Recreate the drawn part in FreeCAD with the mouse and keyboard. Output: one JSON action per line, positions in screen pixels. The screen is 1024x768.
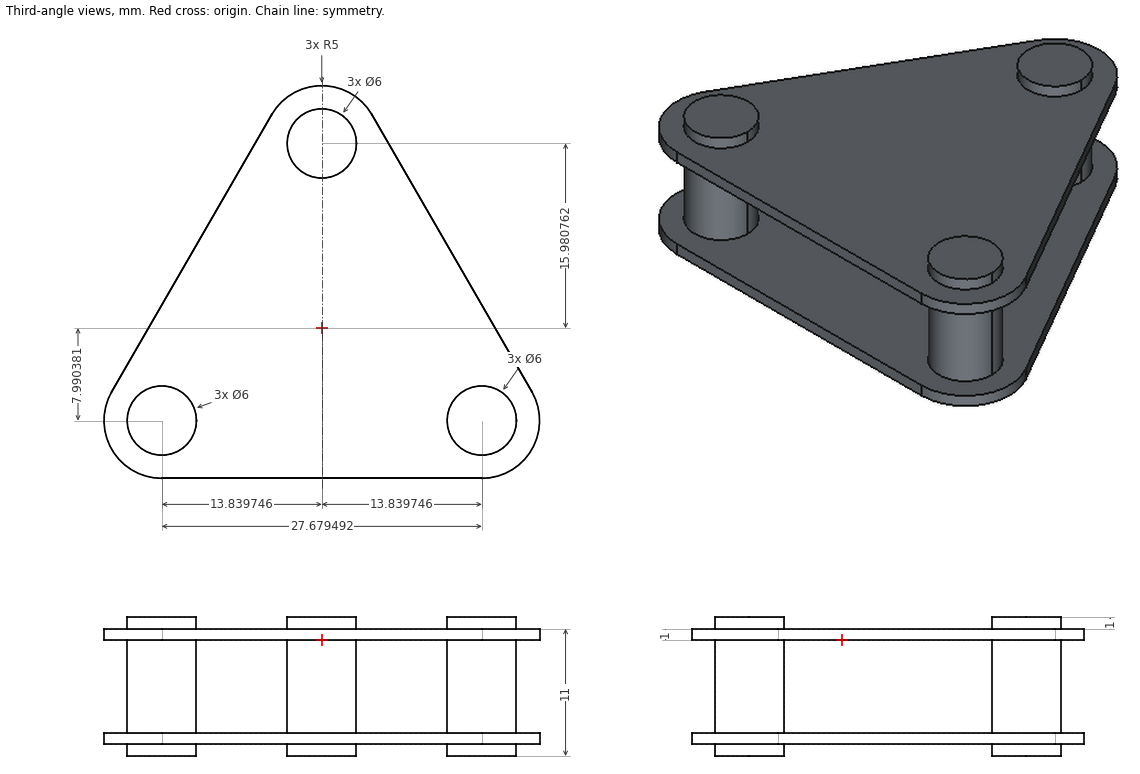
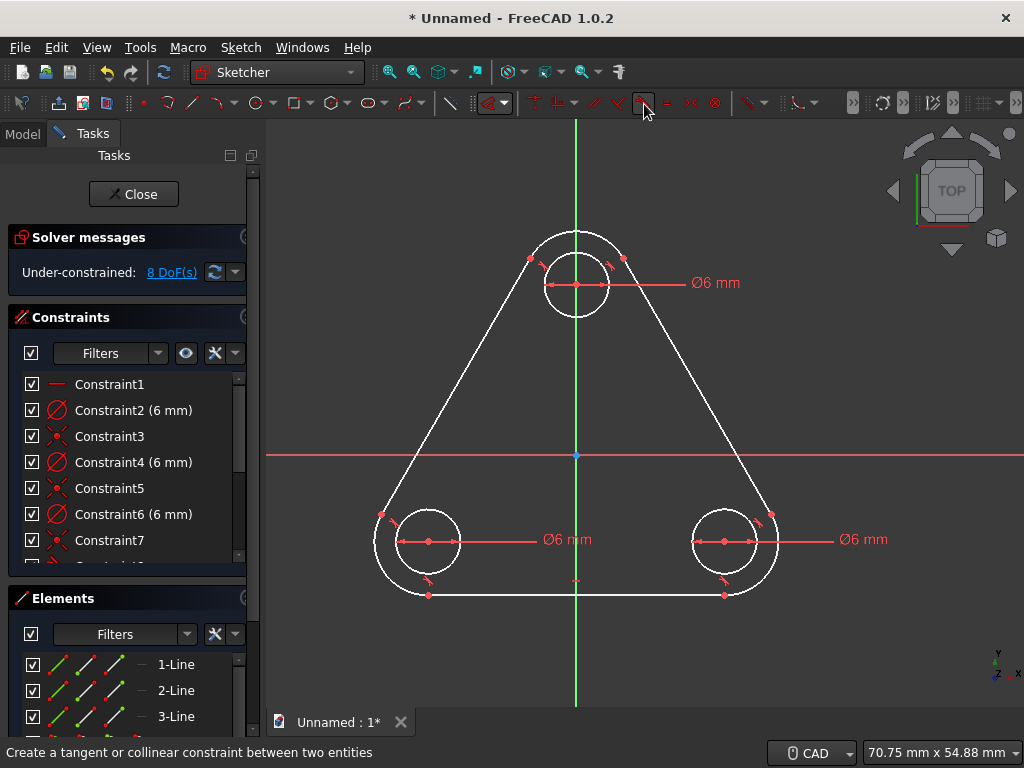
{"action": "left_click", "coordinate": [599, 236]}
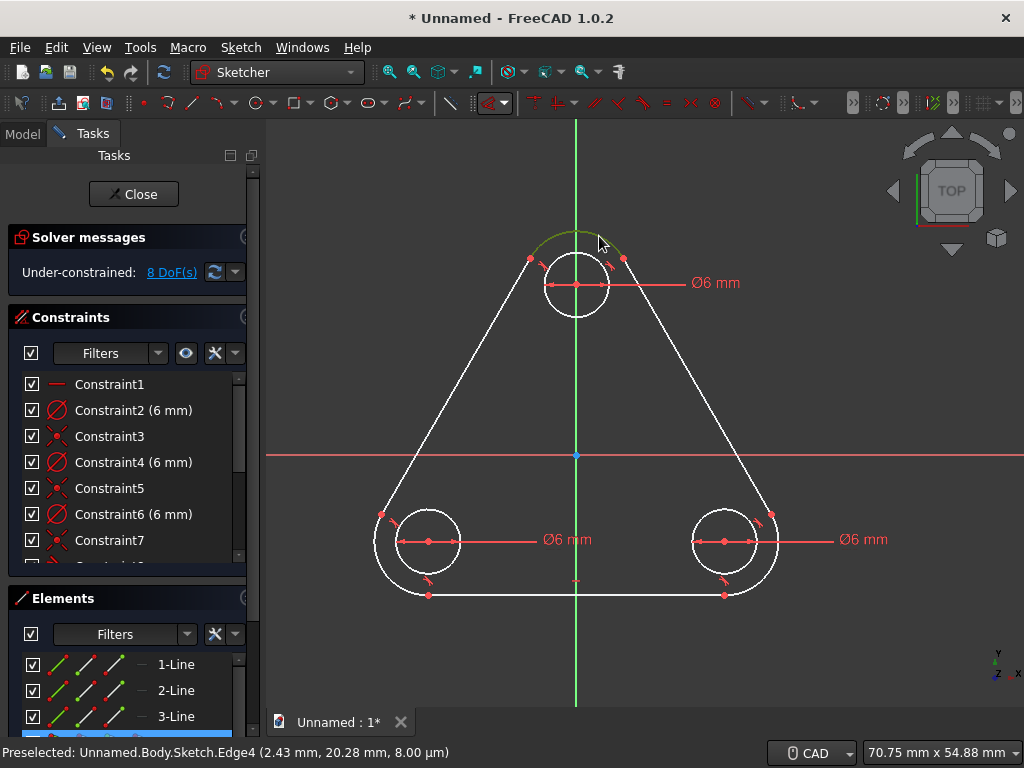
{"action": "left_click", "coordinate": [375, 547]}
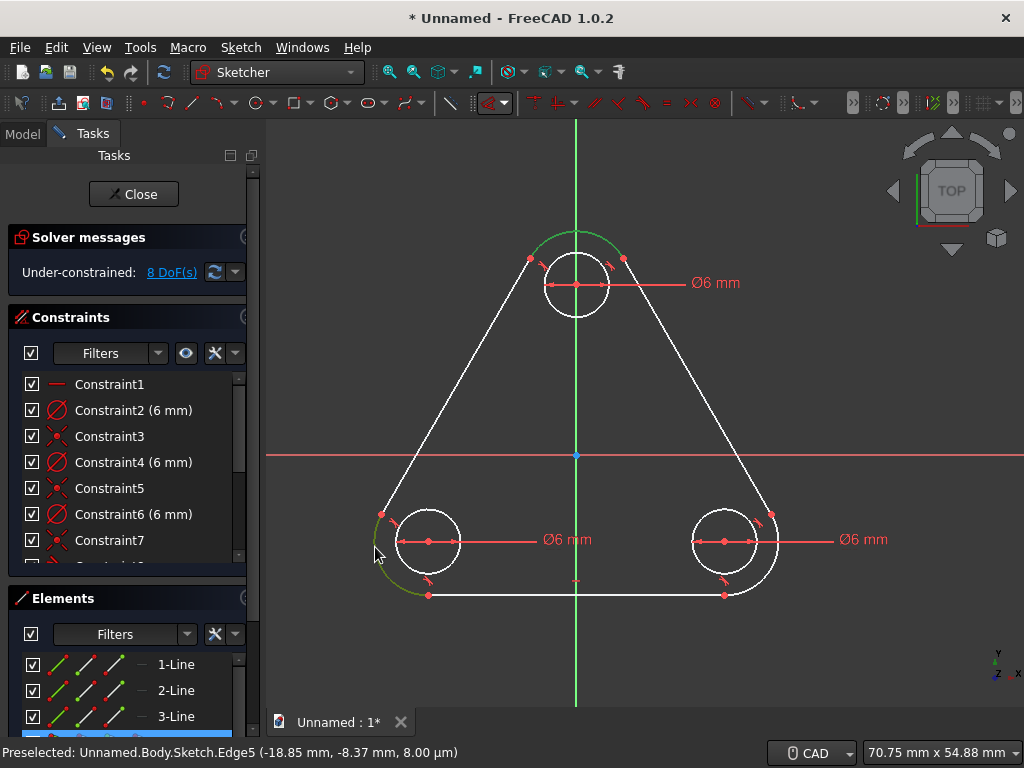
{"action": "left_click", "coordinate": [756, 585]}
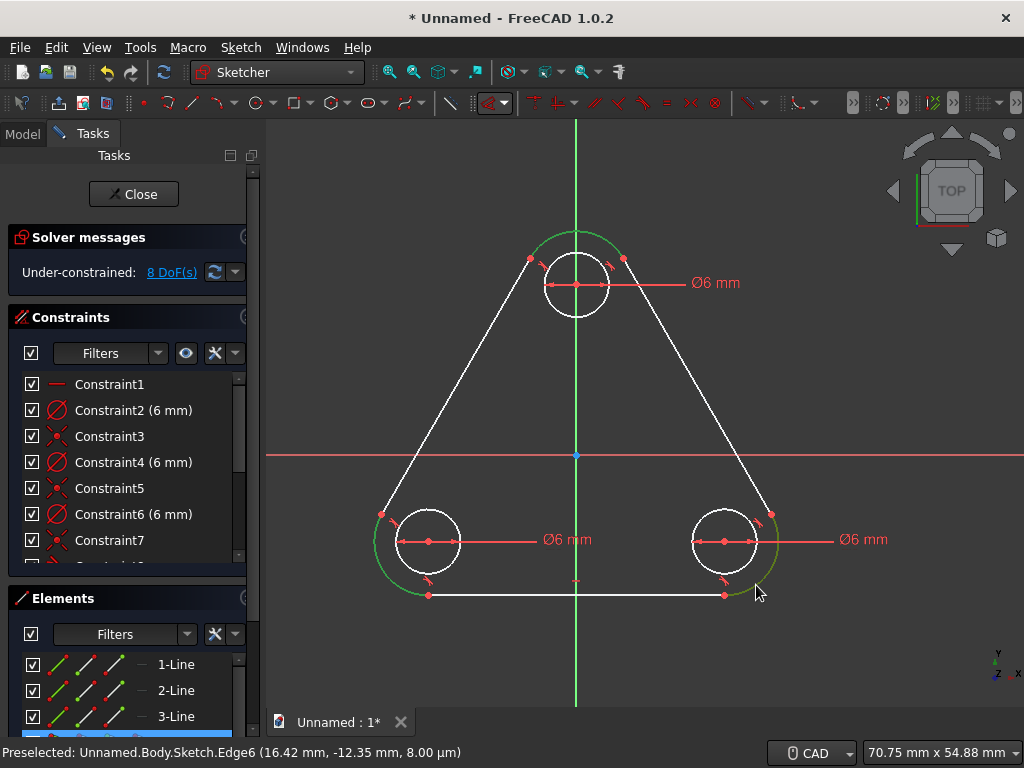
{"action": "left_click", "coordinate": [668, 104]}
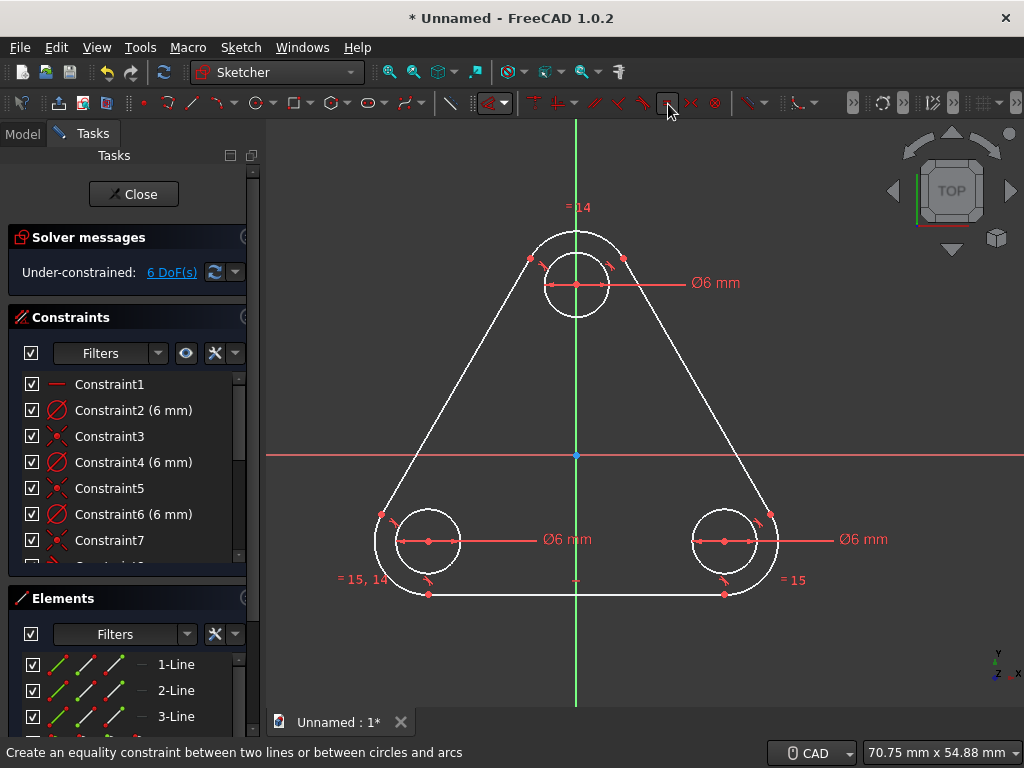
{"action": "left_click", "coordinate": [577, 285]}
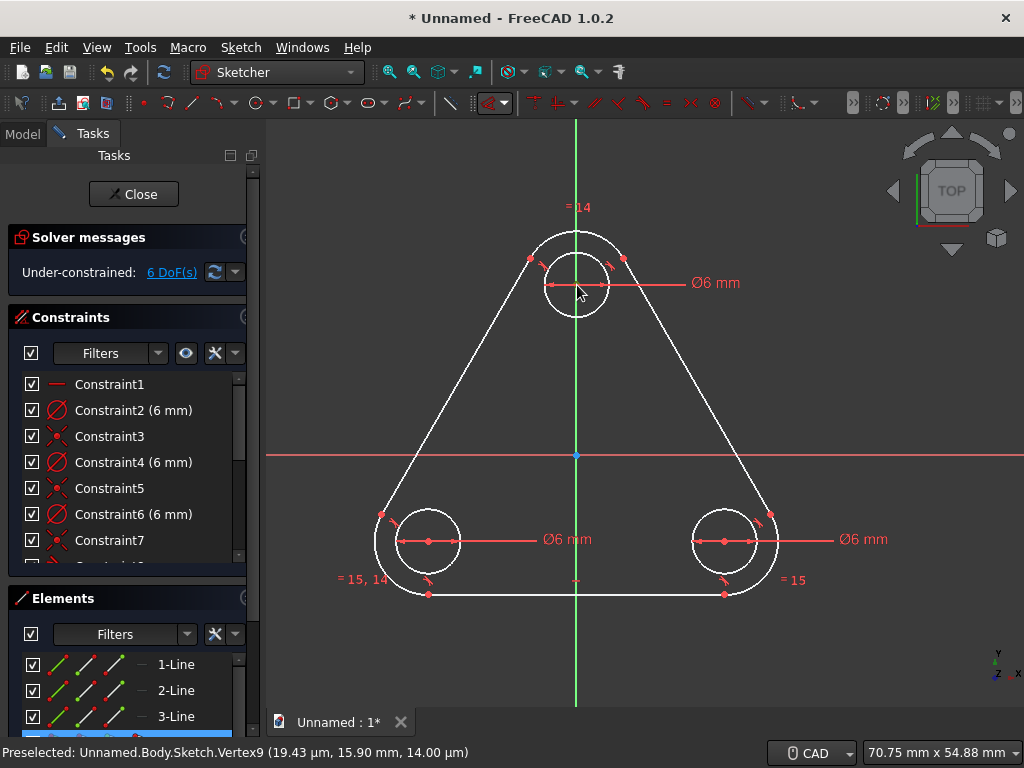
{"action": "left_click", "coordinate": [576, 641]}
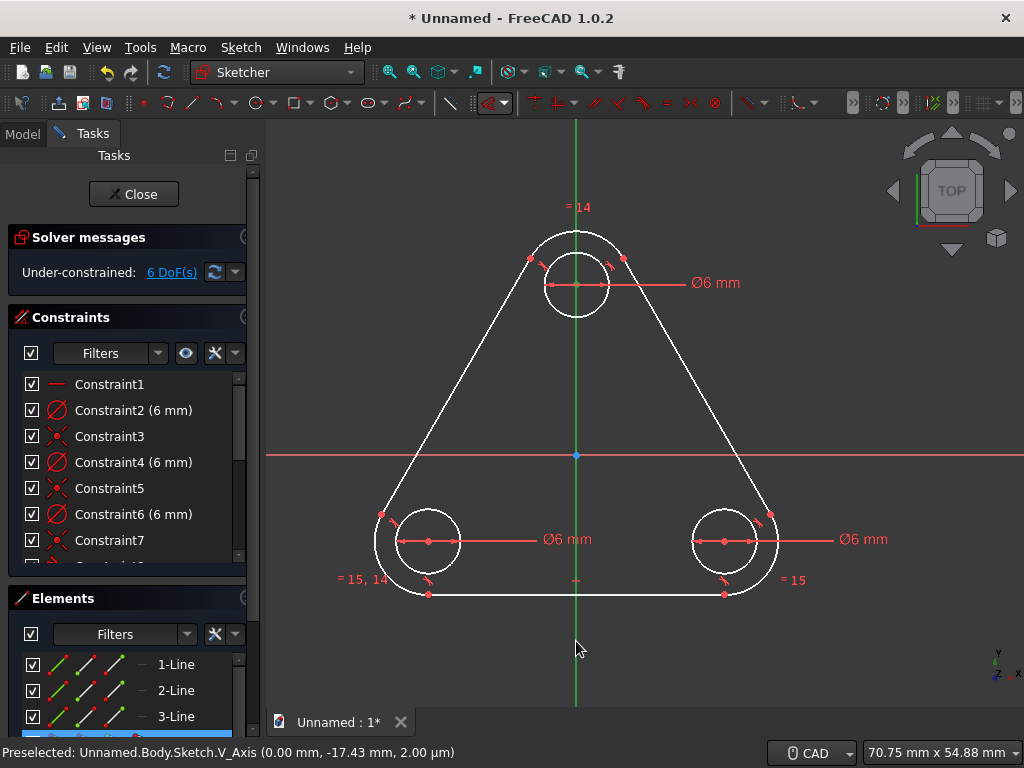
{"action": "left_click", "coordinate": [534, 104]}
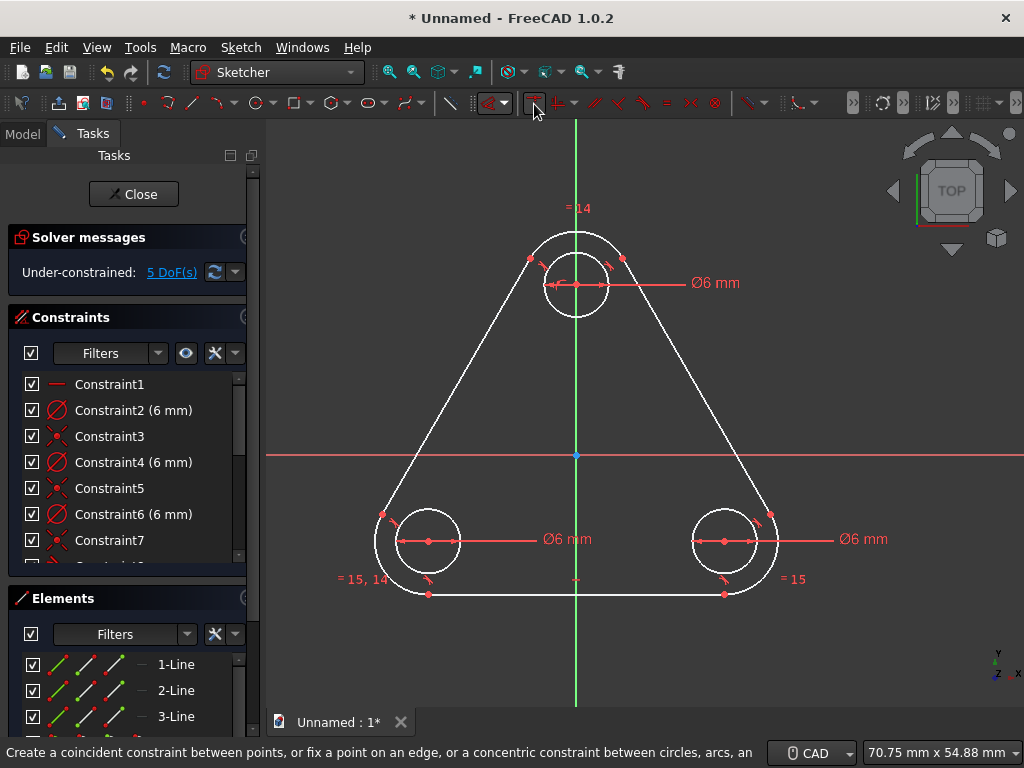
{"action": "left_click", "coordinate": [598, 236]}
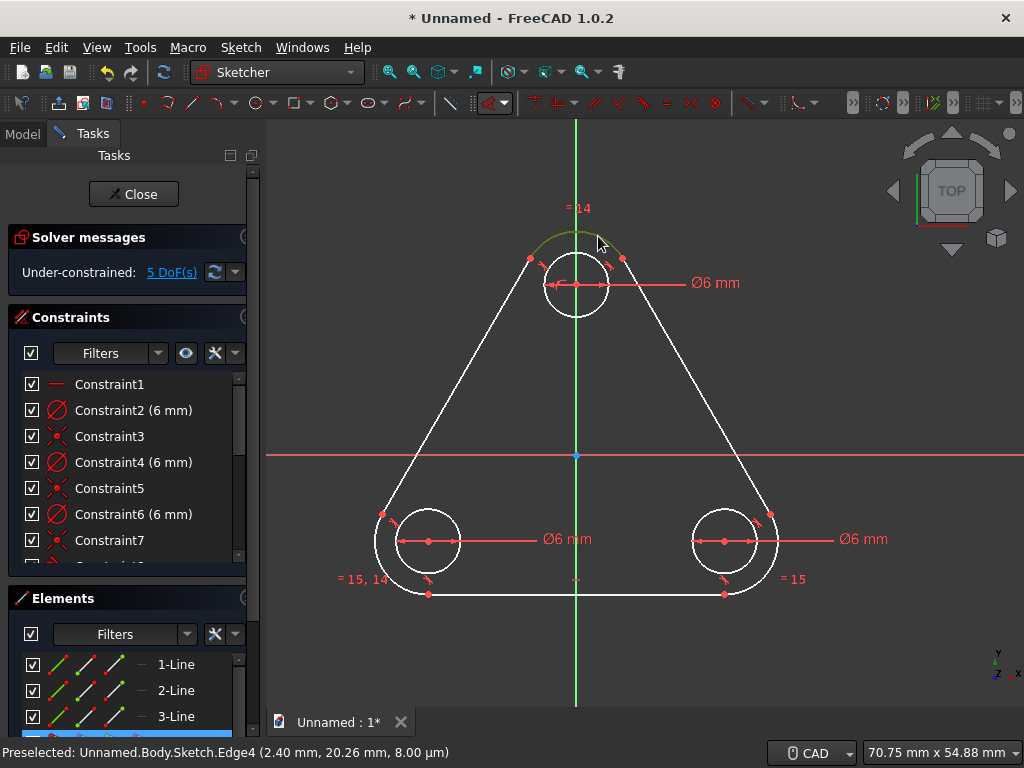
{"action": "left_click", "coordinate": [506, 104]}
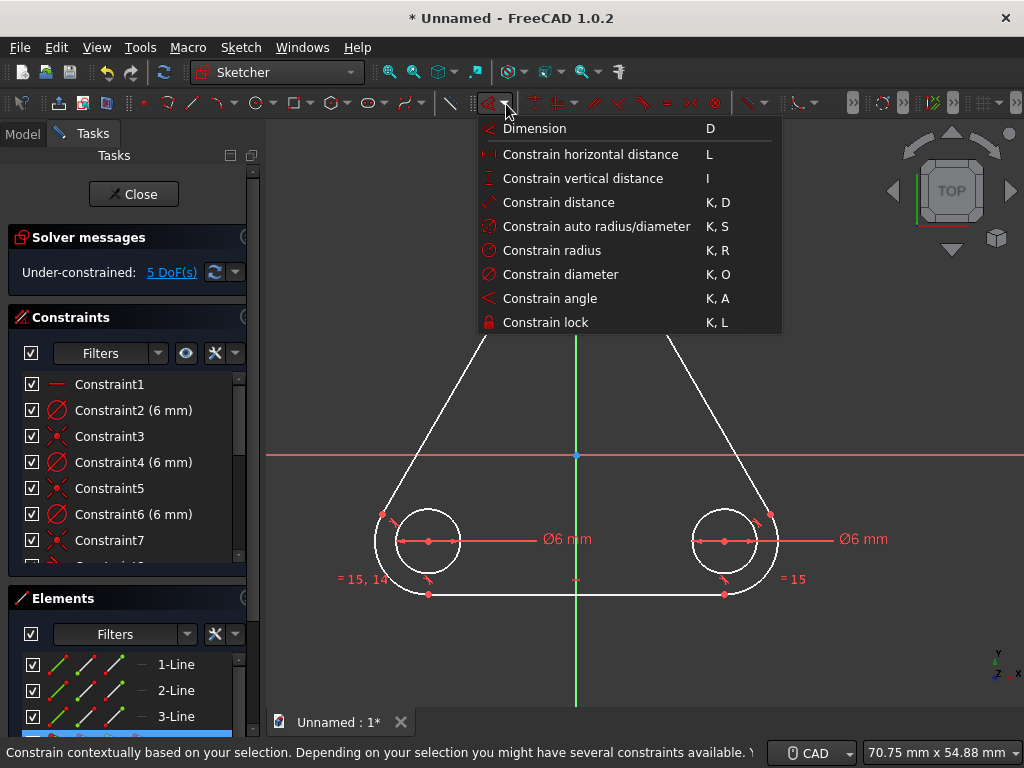
{"action": "left_click", "coordinate": [630, 250]}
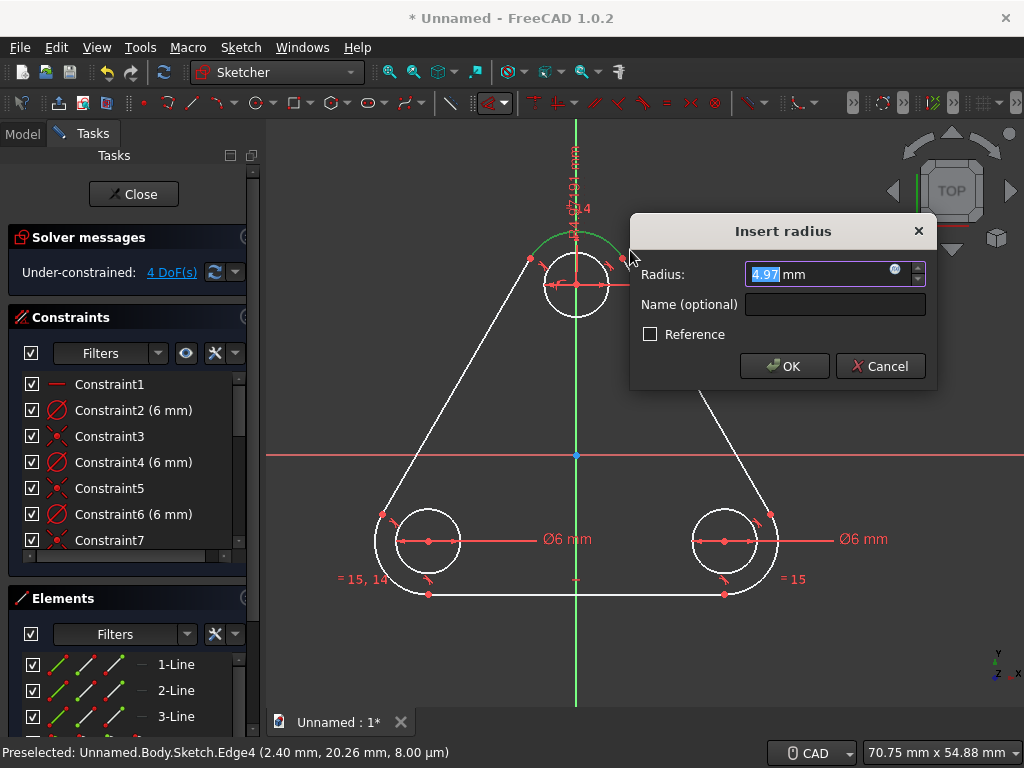
{"action": "type", "text": "5"}
{"action": "key", "text": "Return"}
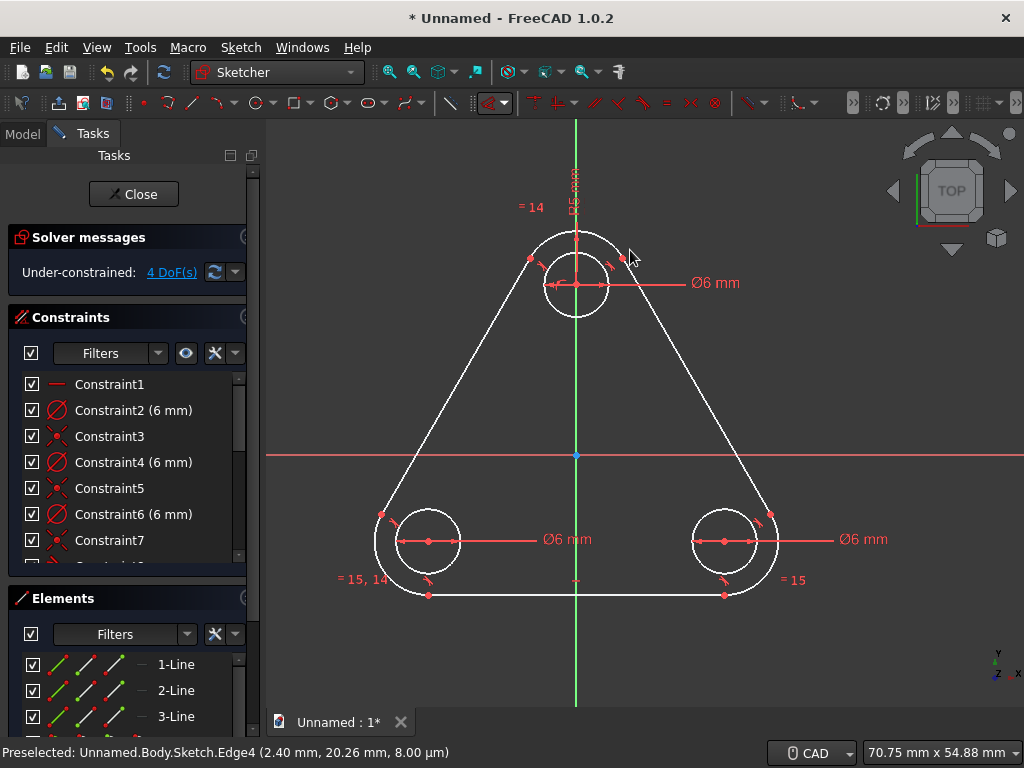
{"action": "left_click", "coordinate": [428, 541]}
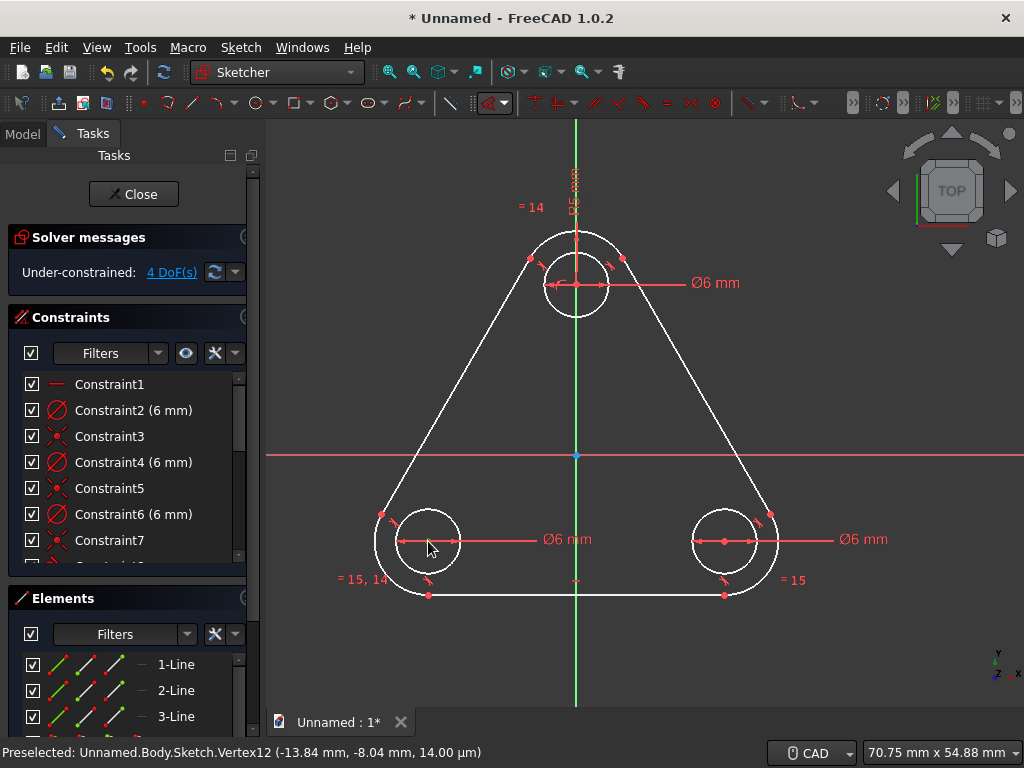
{"action": "left_click", "coordinate": [506, 104]}